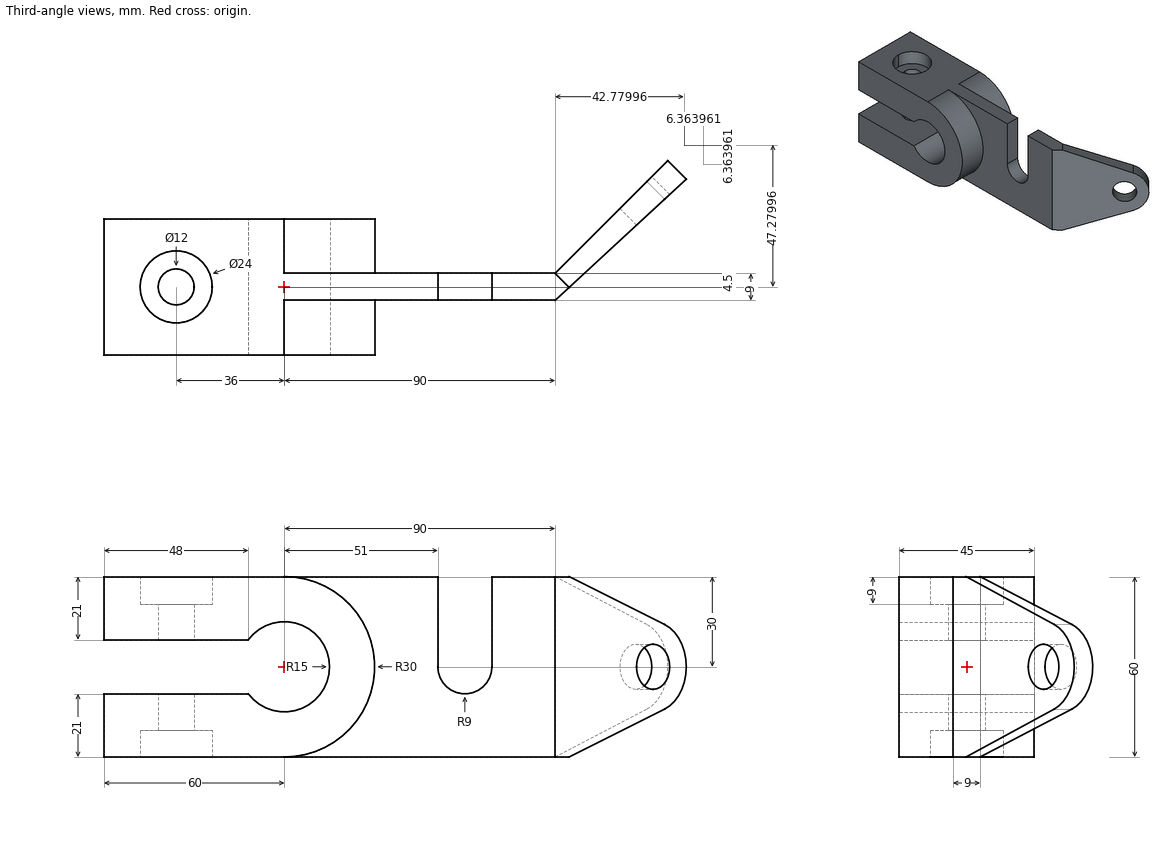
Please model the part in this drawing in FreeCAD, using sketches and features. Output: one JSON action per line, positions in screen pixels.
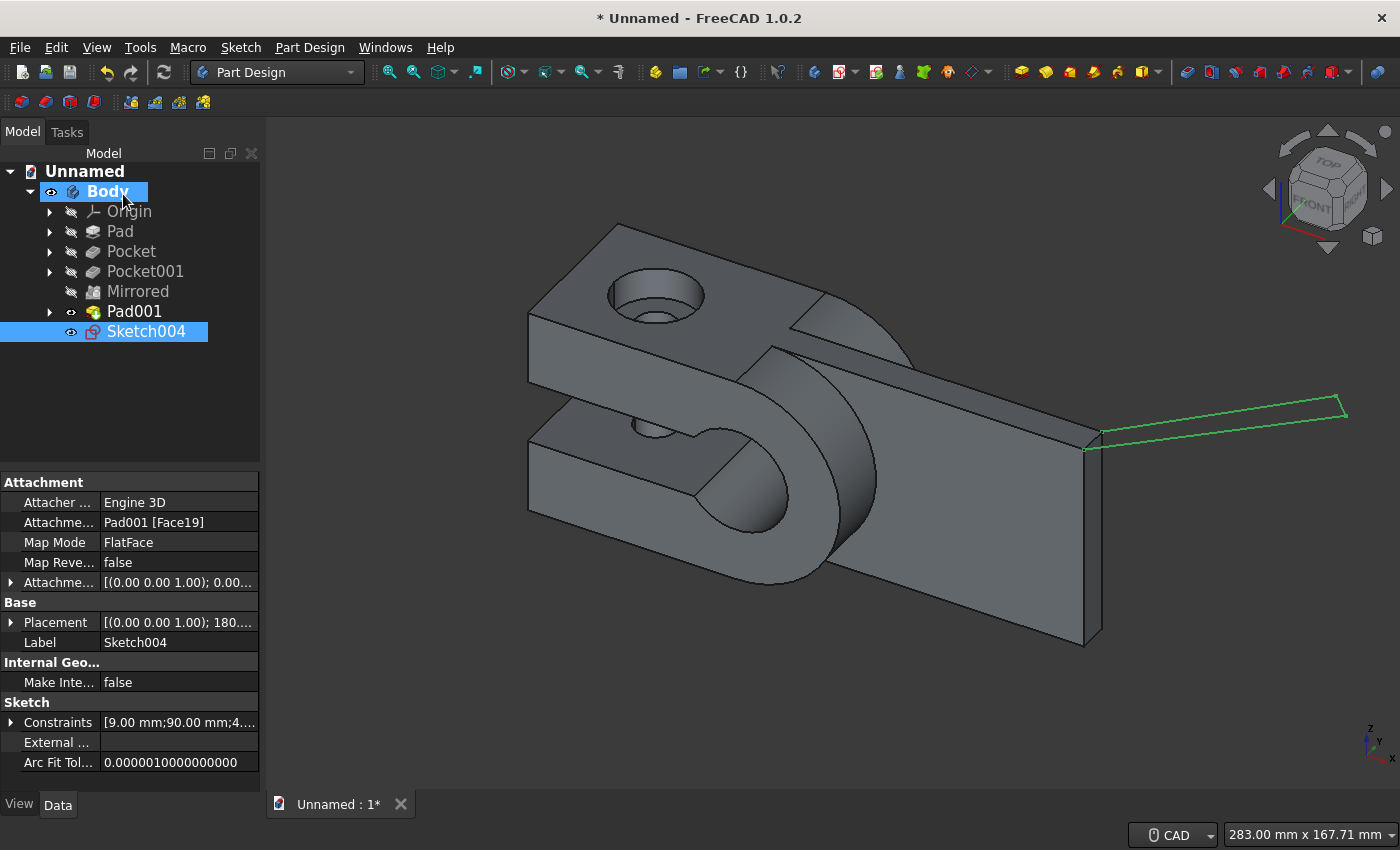
{"action": "left_click", "coordinate": [1022, 72]}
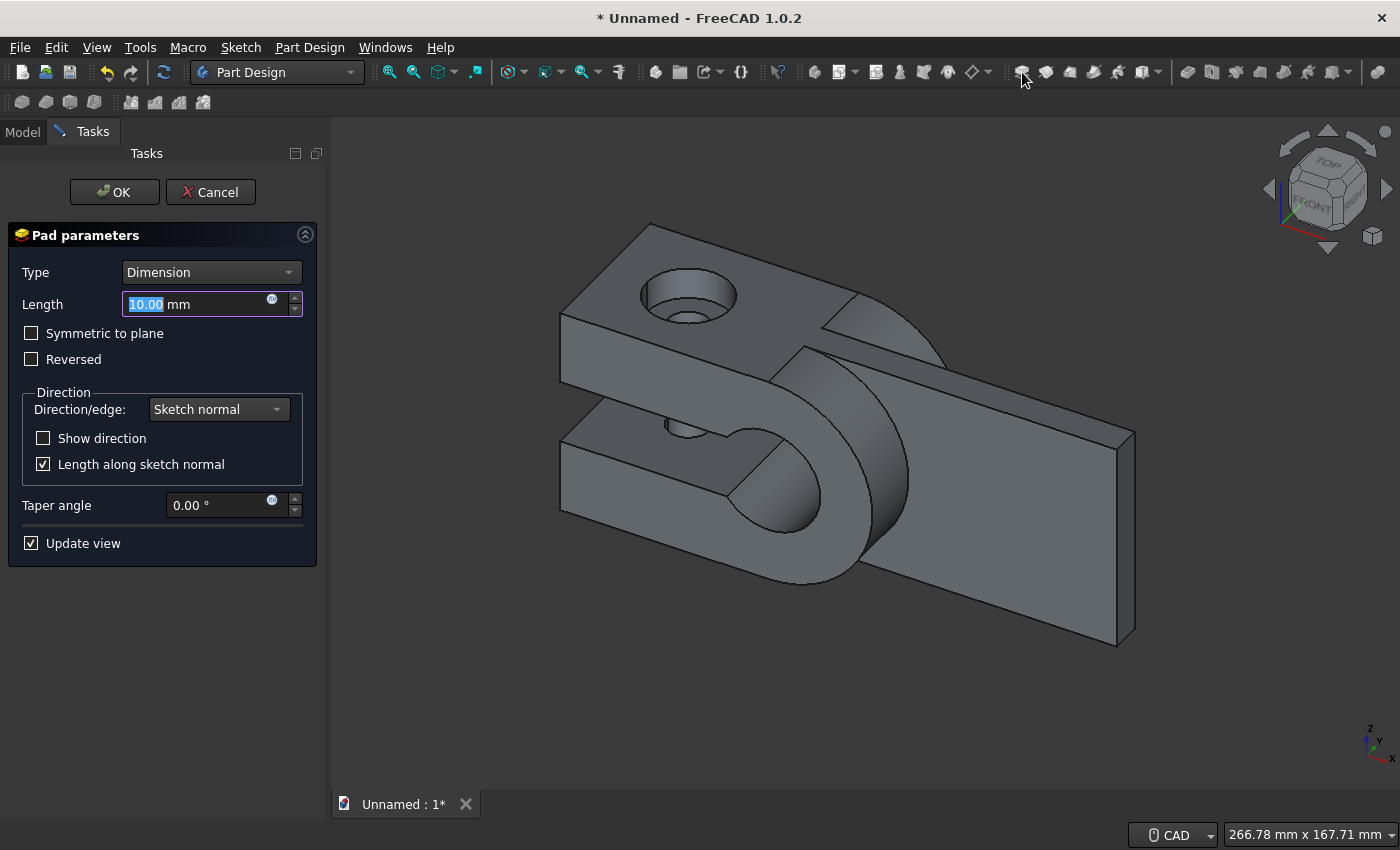
{"action": "type", "text": "60"}
{"action": "key", "text": "Tab"}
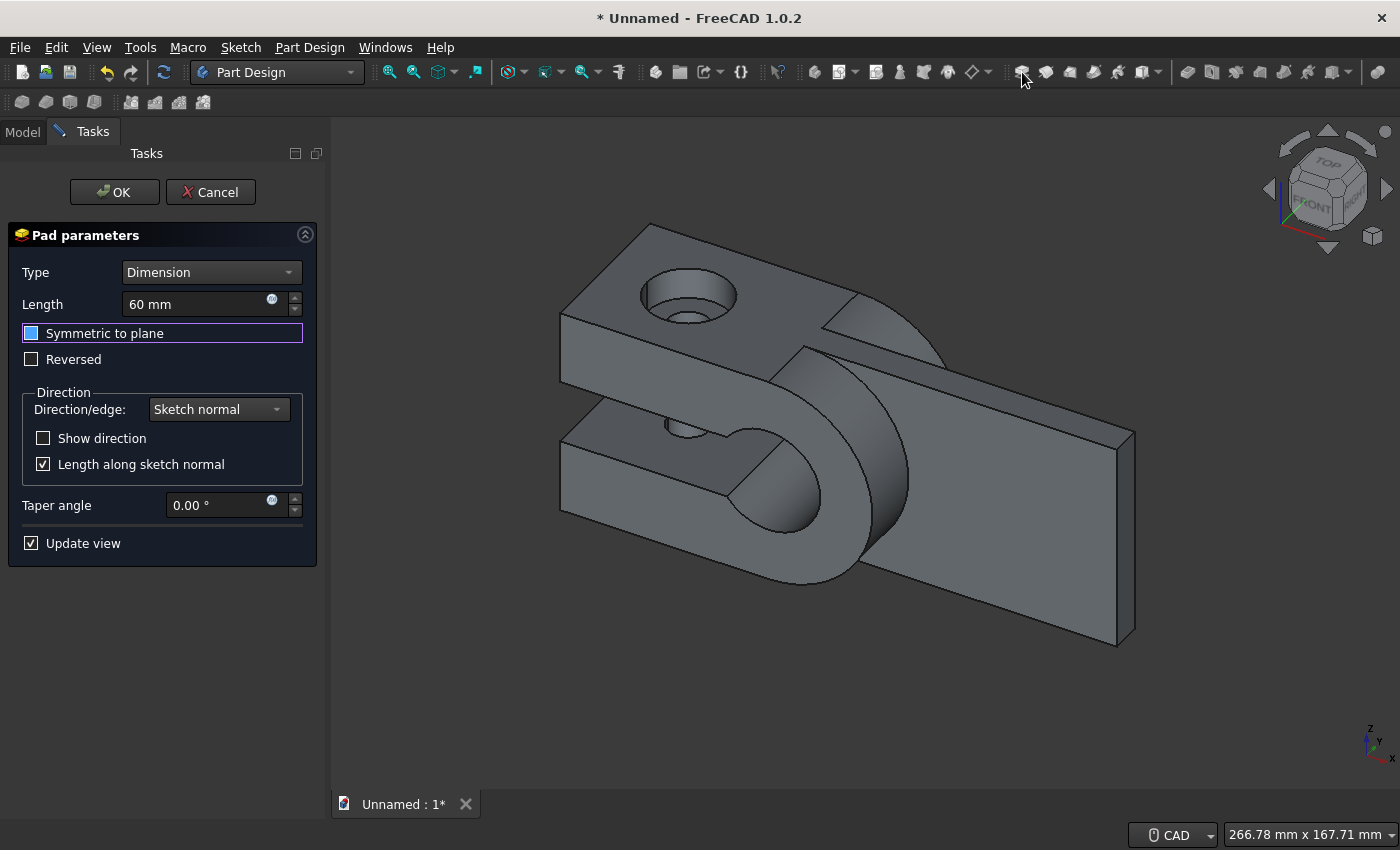
{"action": "left_click", "coordinate": [30, 359]}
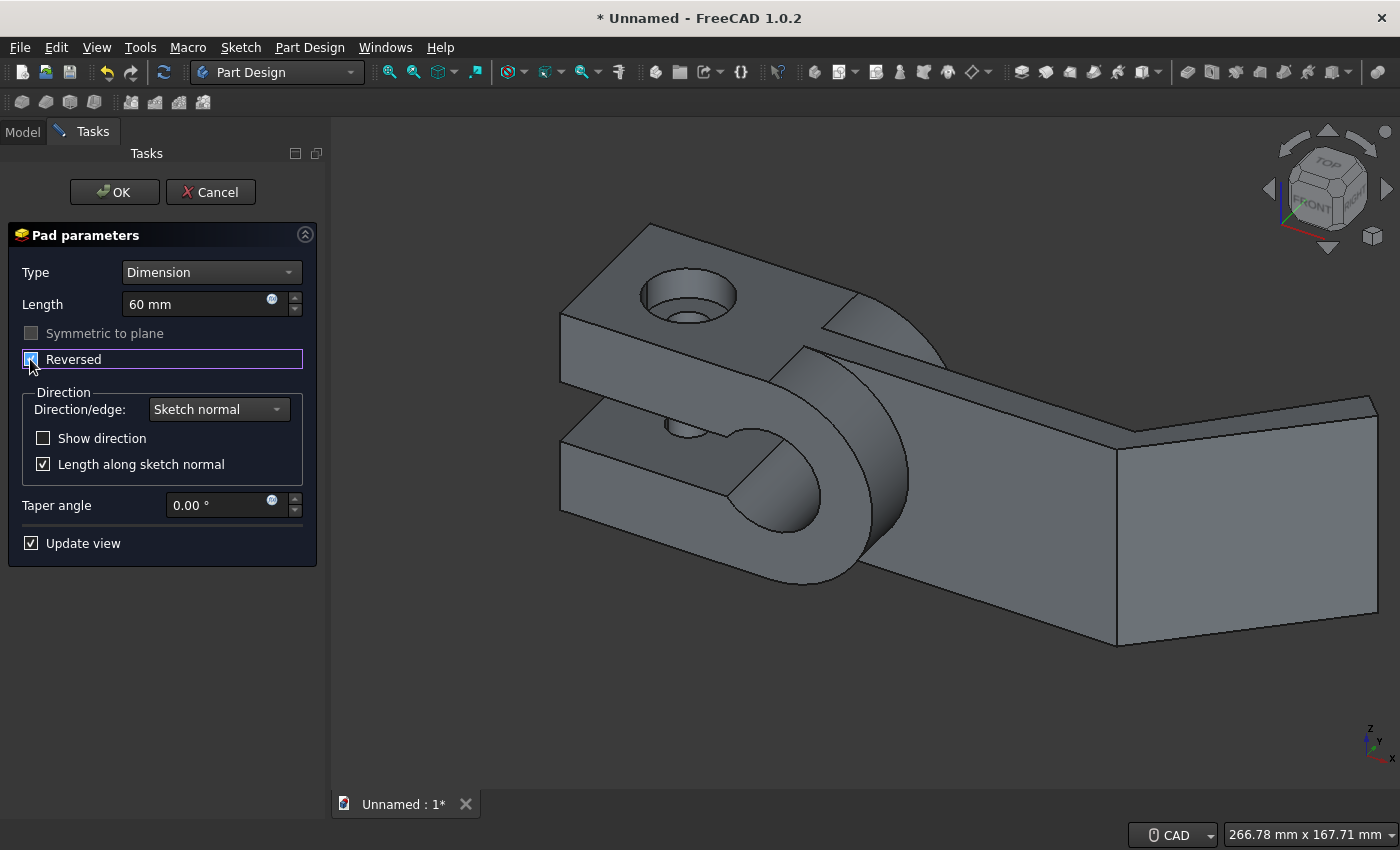
{"action": "left_click", "coordinate": [115, 192]}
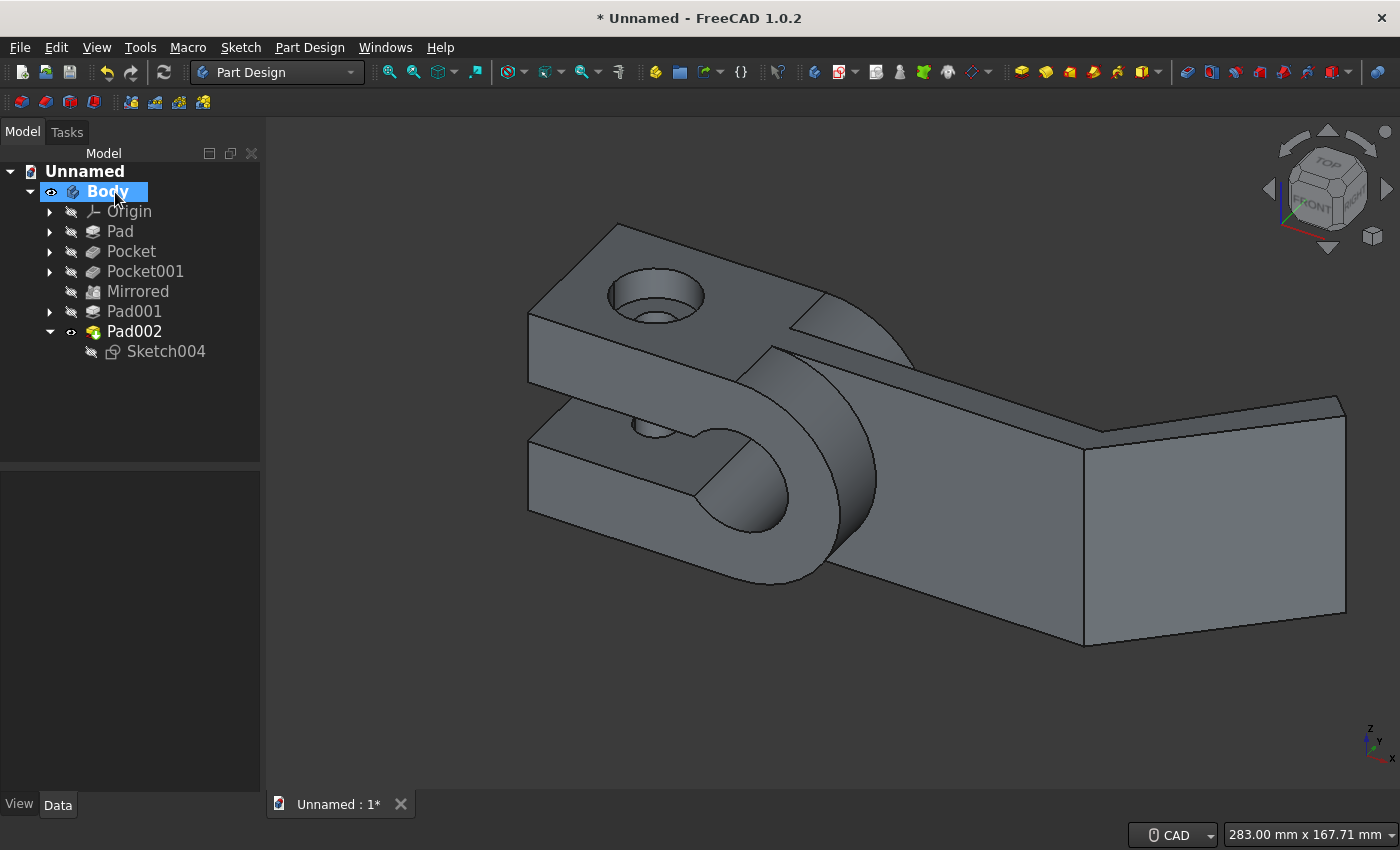
{"action": "key", "text": "4"}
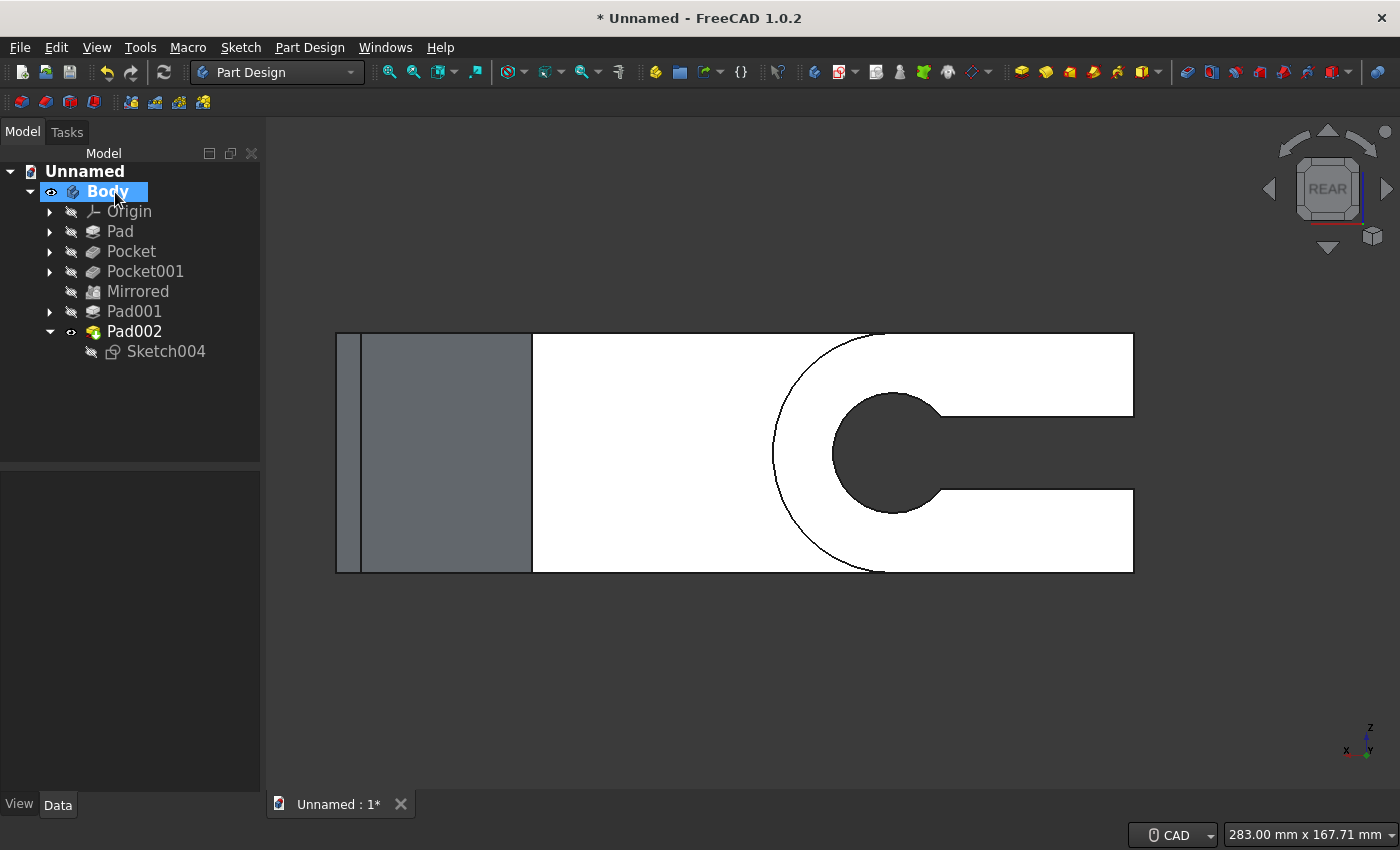
{"action": "left_click", "coordinate": [661, 452]}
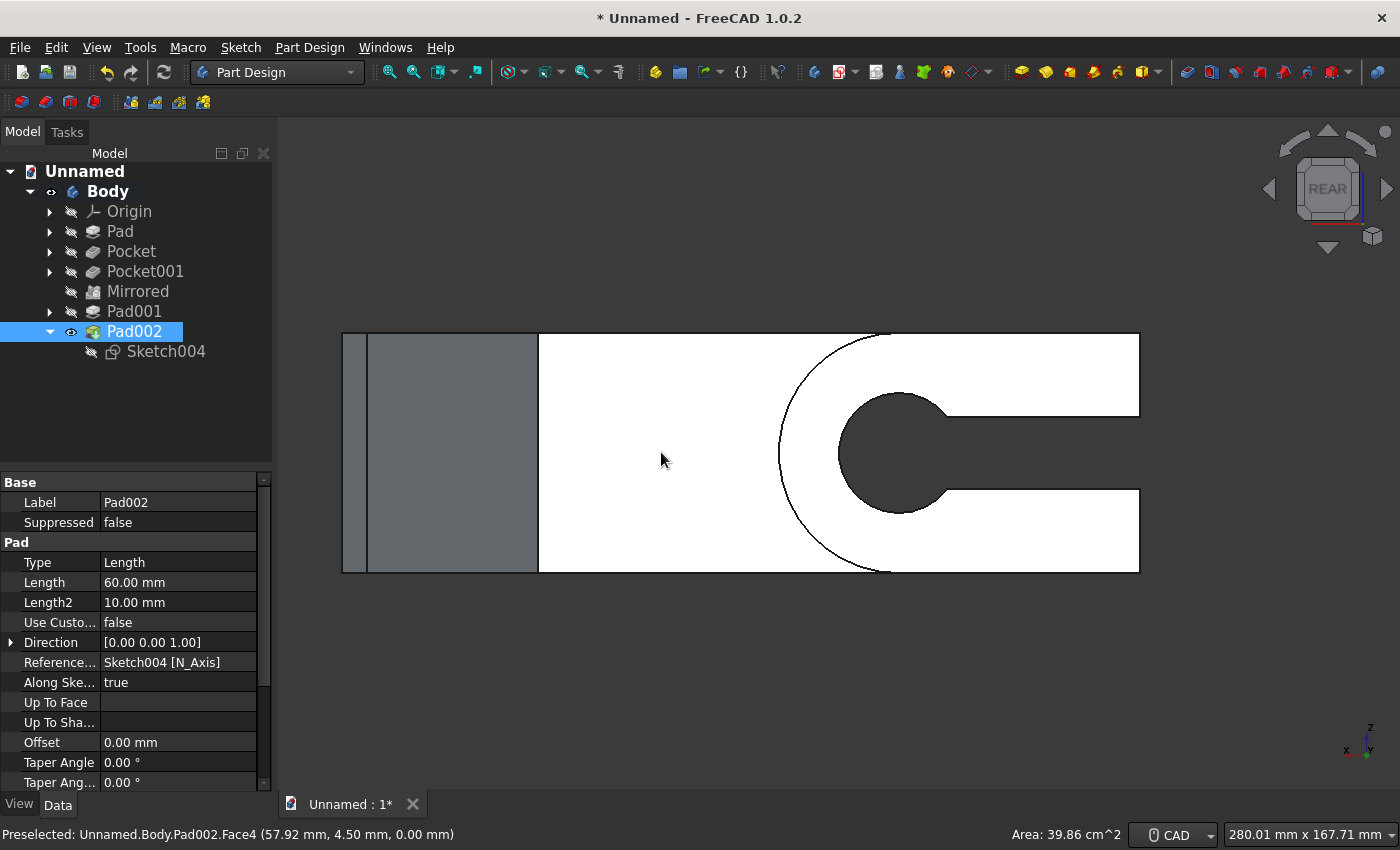
{"action": "left_click", "coordinate": [840, 72]}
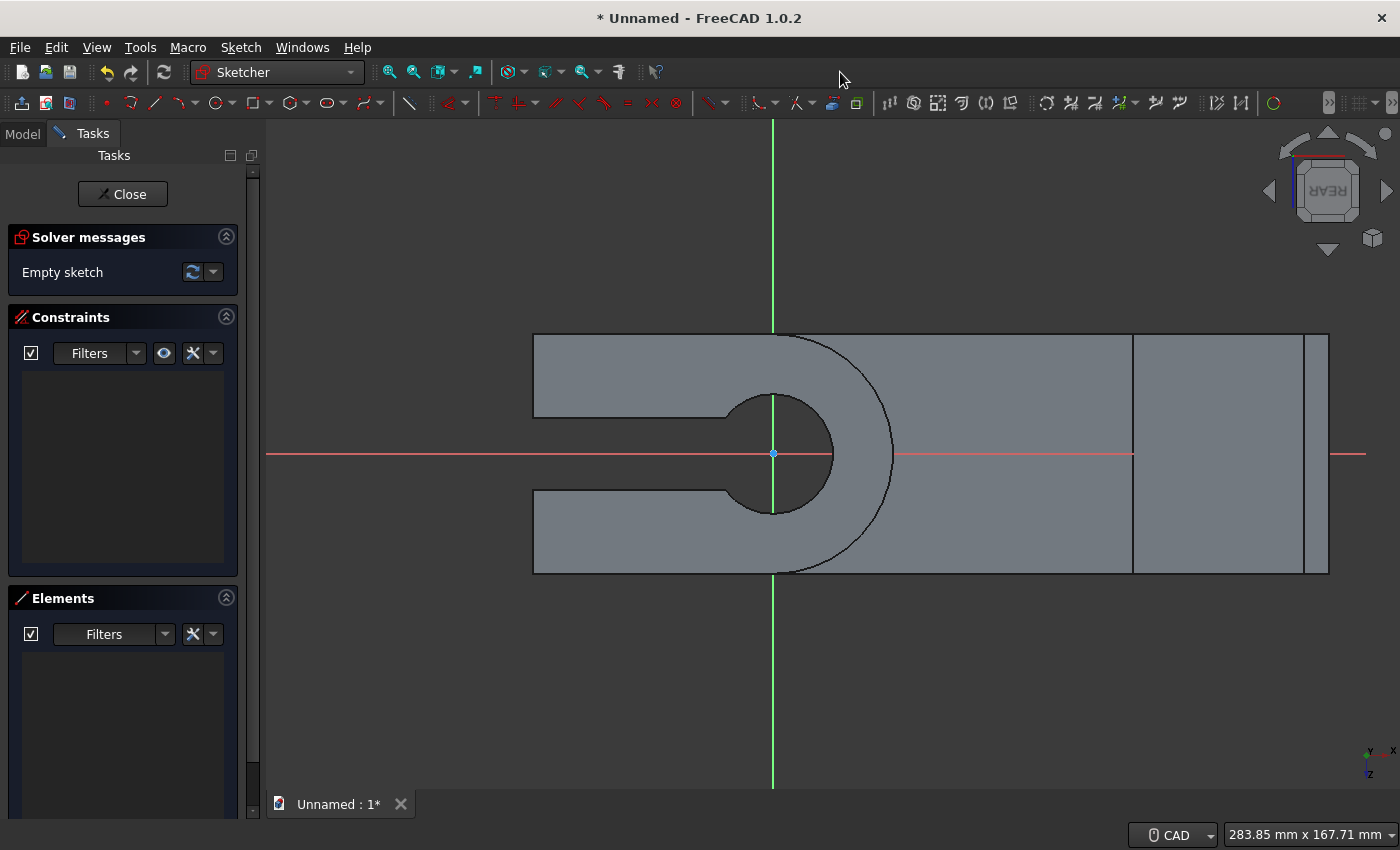
{"action": "scroll", "coordinate": [1030, 530], "scroll_direction": "up", "scroll_amount": 4}